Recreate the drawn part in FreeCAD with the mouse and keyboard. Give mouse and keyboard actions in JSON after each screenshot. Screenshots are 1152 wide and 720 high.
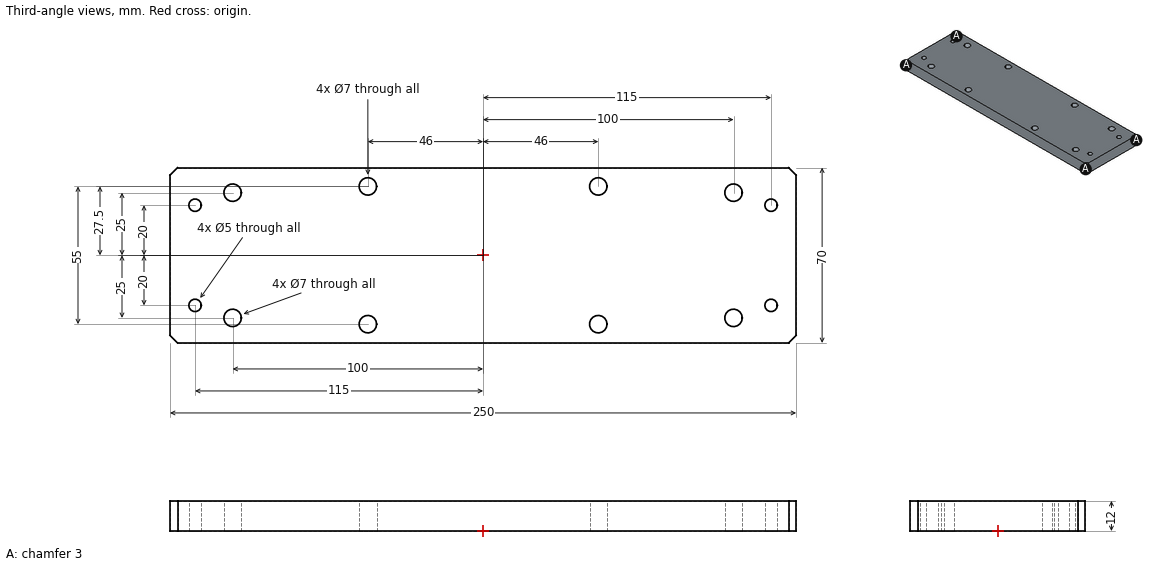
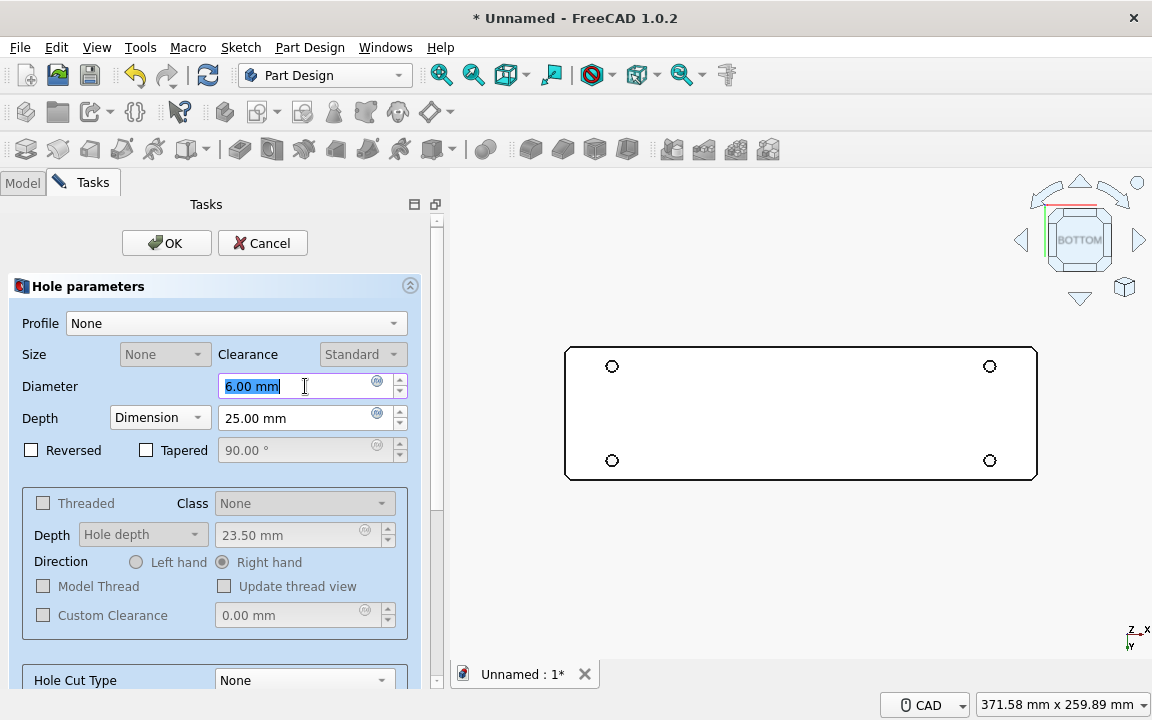
{"action": "type", "text": "7"}
{"action": "key", "text": "Tab"}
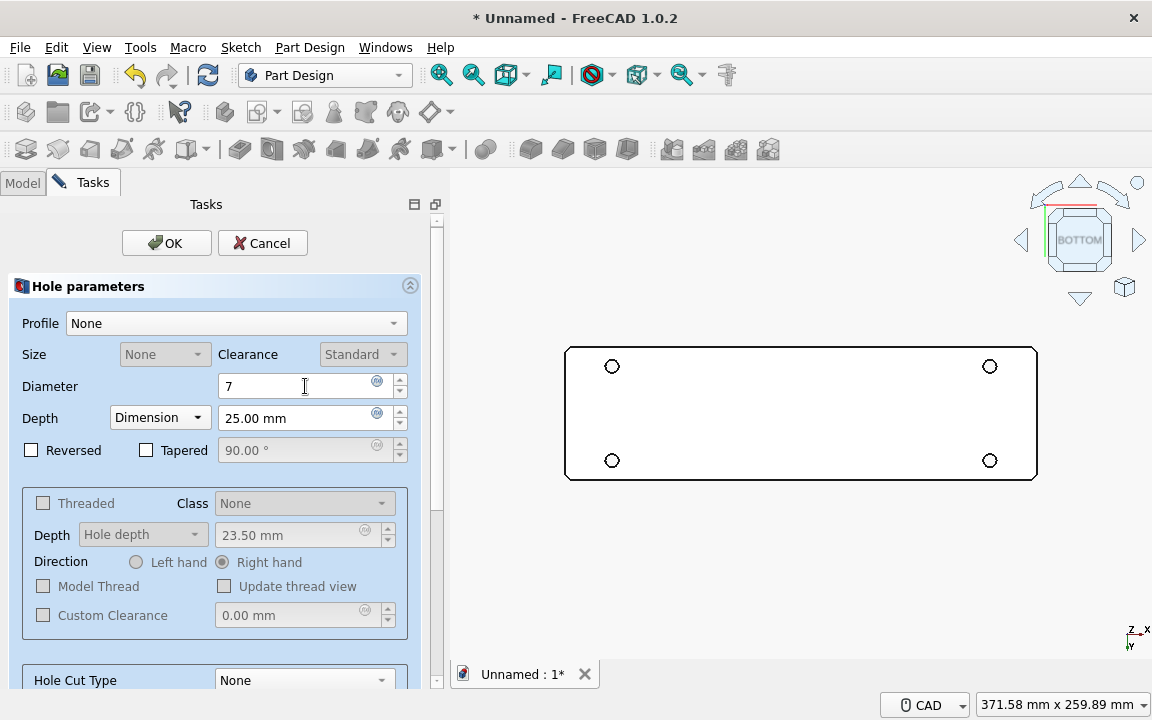
{"action": "left_click", "coordinate": [161, 418]}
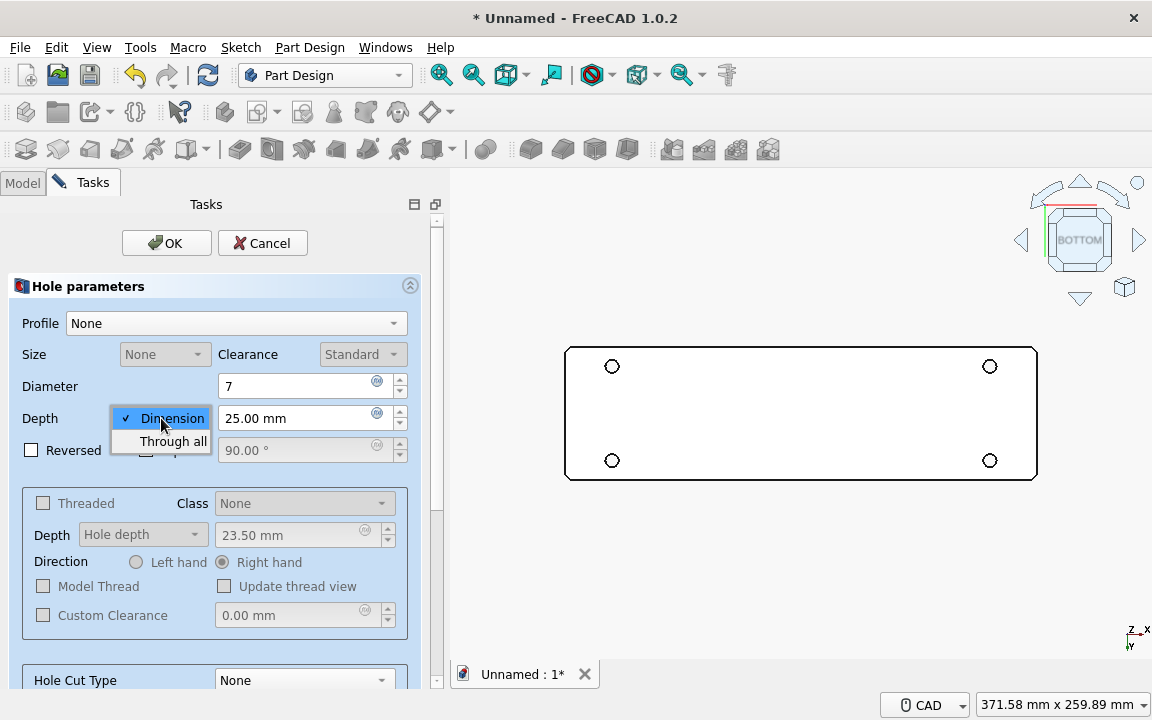
{"action": "left_click", "coordinate": [160, 442]}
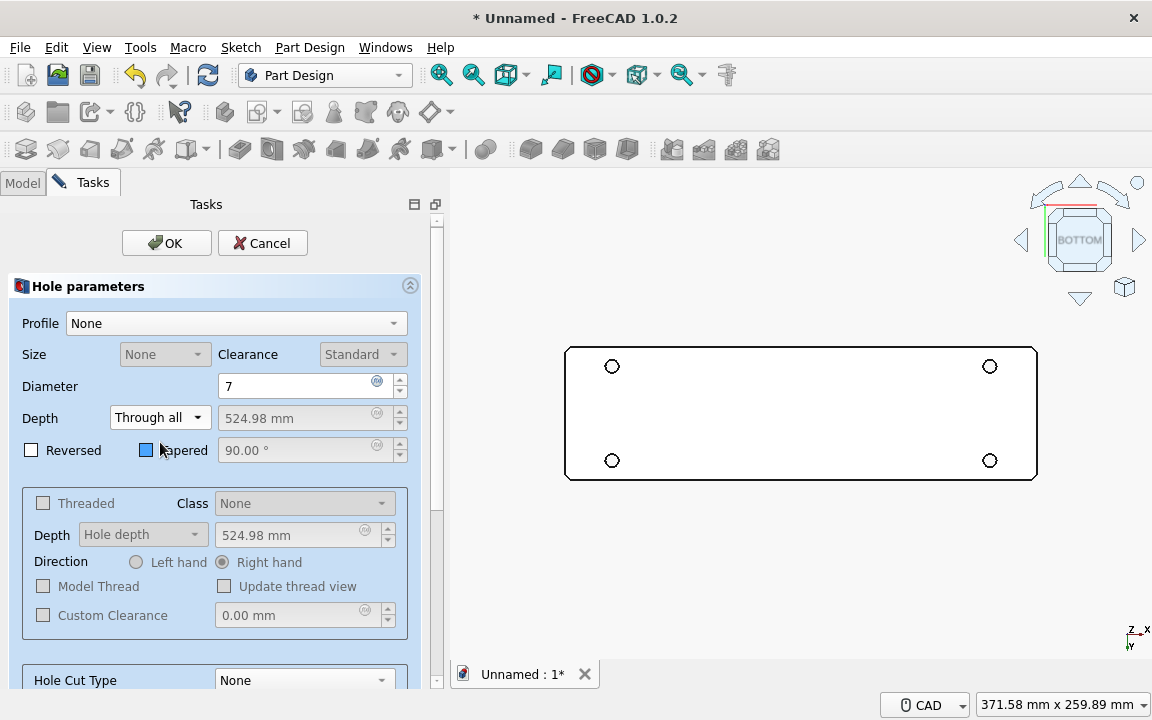
{"action": "left_click", "coordinate": [167, 243]}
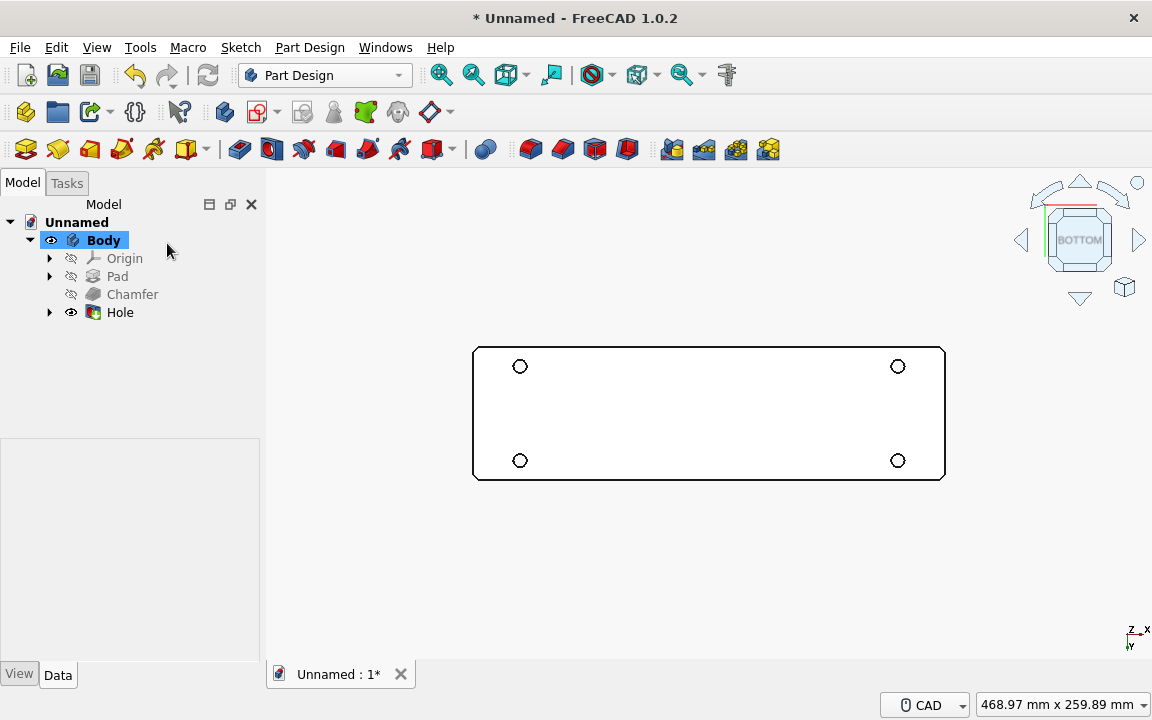
{"action": "left_click", "coordinate": [776, 412]}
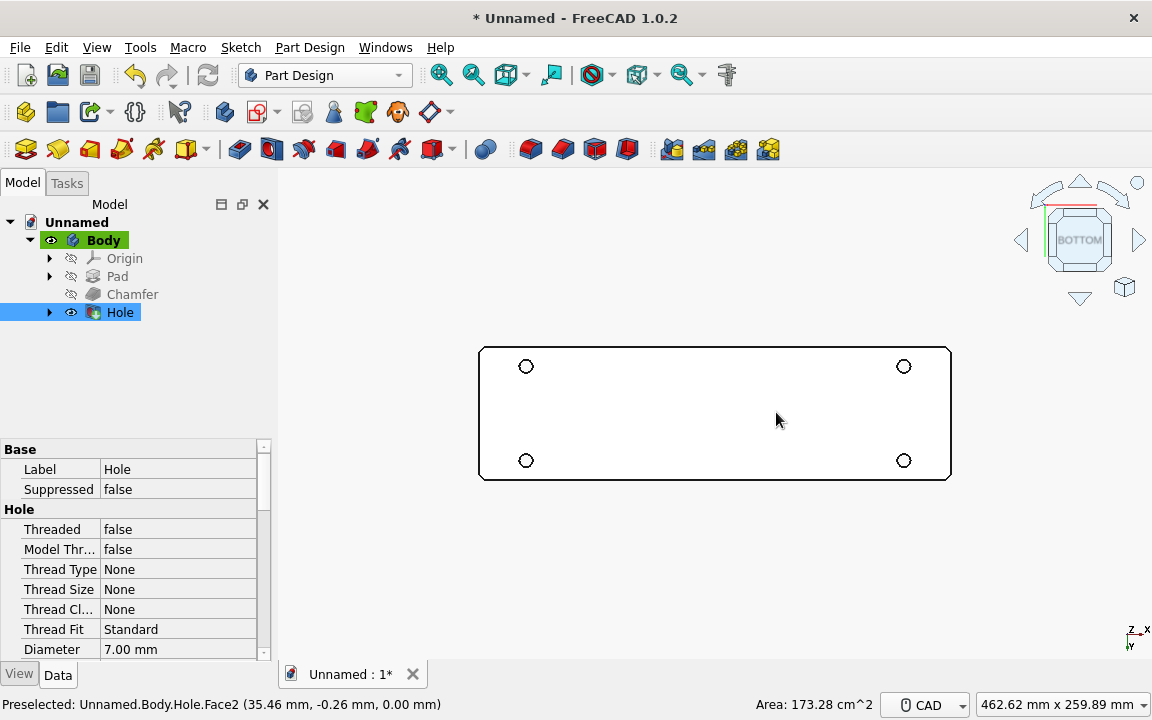
{"action": "left_click", "coordinate": [258, 112]}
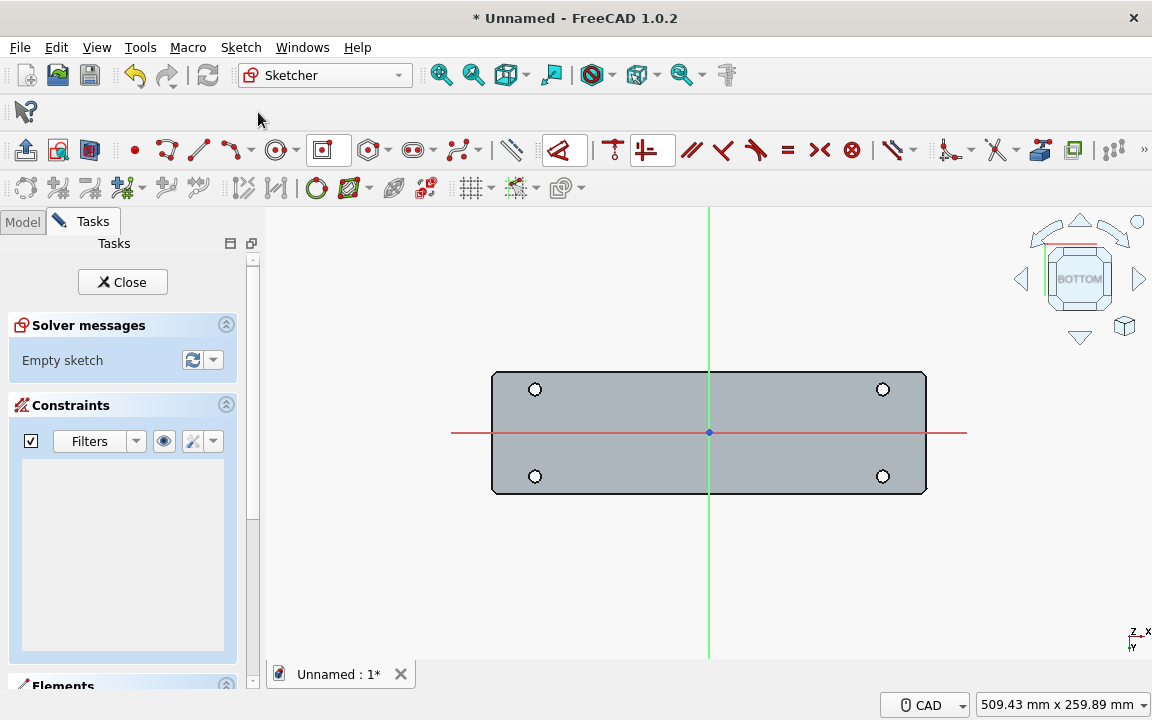
{"action": "left_click", "coordinate": [276, 150]}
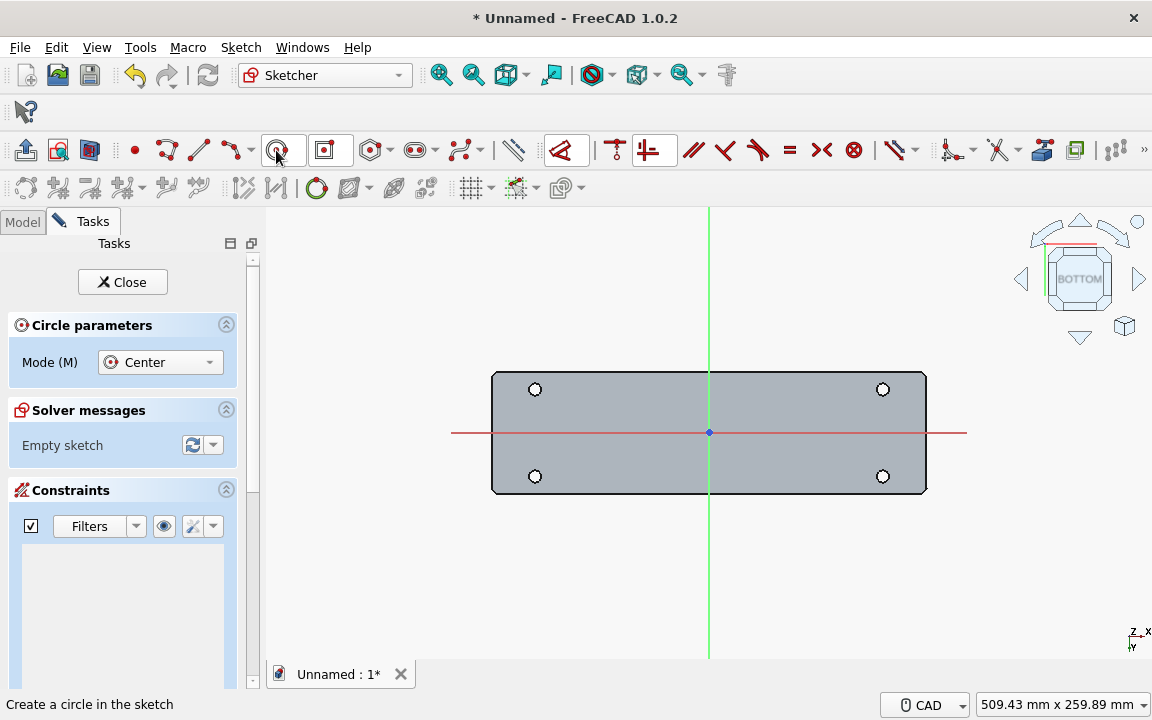
{"action": "scroll", "coordinate": [509, 398], "scroll_direction": "up", "scroll_amount": 9}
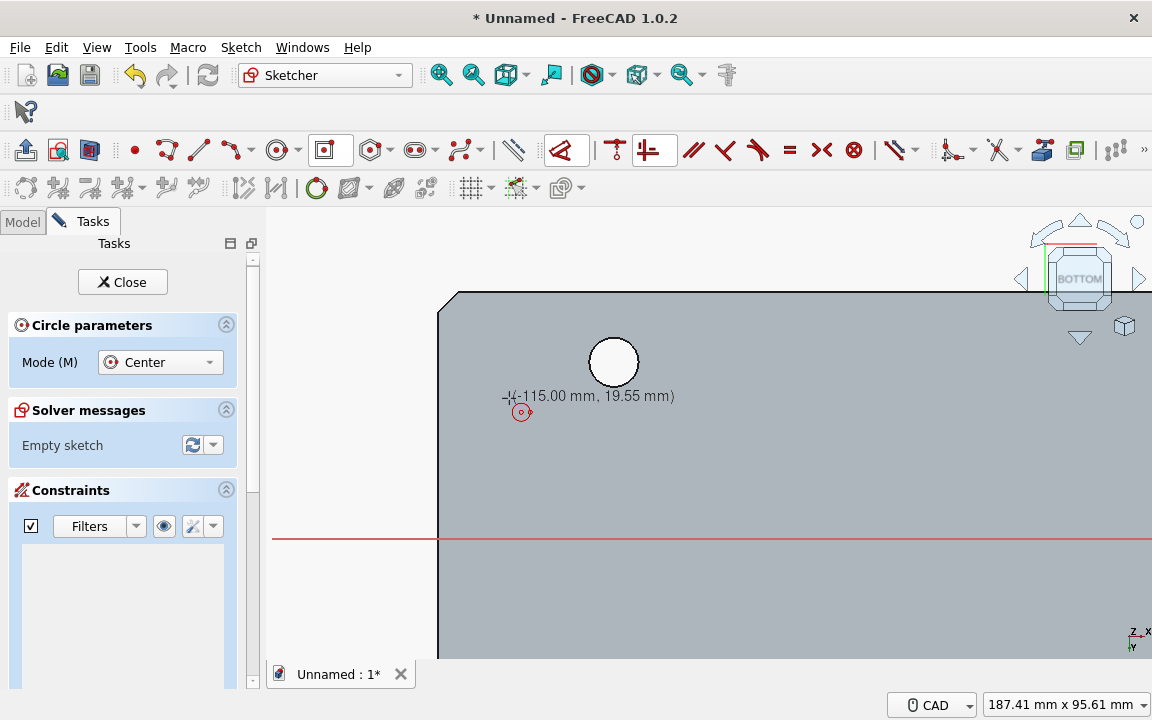
{"action": "scroll", "coordinate": [368, 389], "scroll_direction": "down", "scroll_amount": 8}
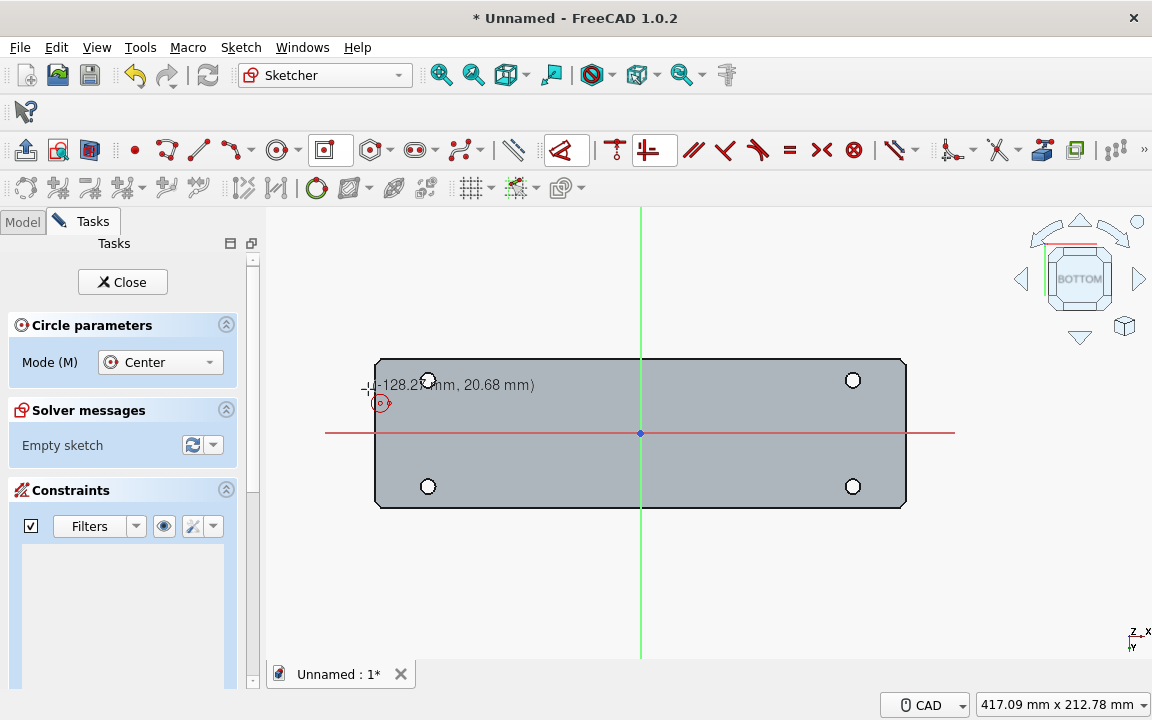
{"action": "left_click", "coordinate": [396, 391]}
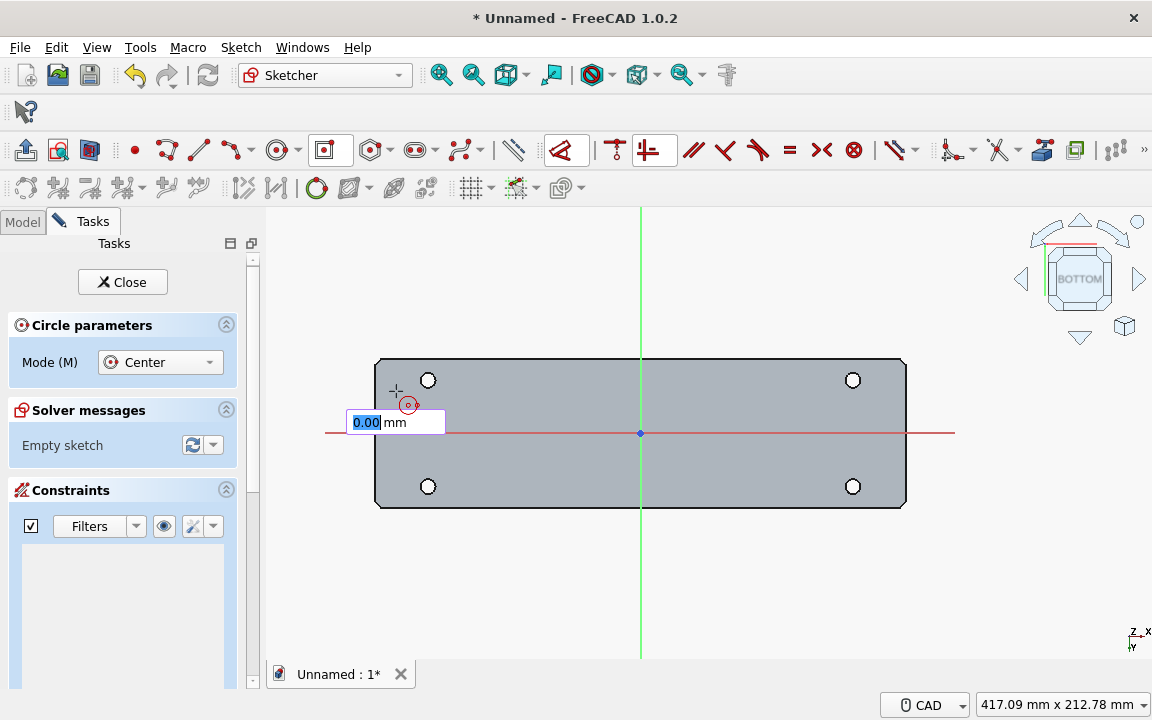
{"action": "scroll", "coordinate": [400, 387], "scroll_direction": "up", "scroll_amount": 6}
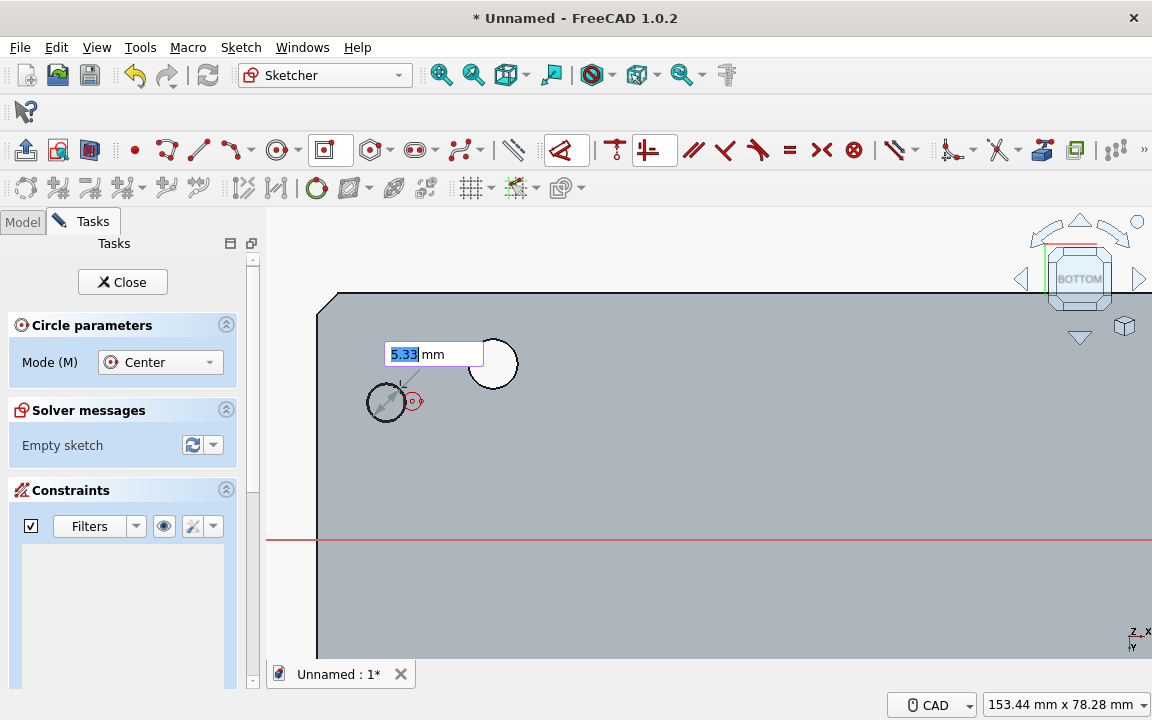
{"action": "left_click", "coordinate": [400, 387]}